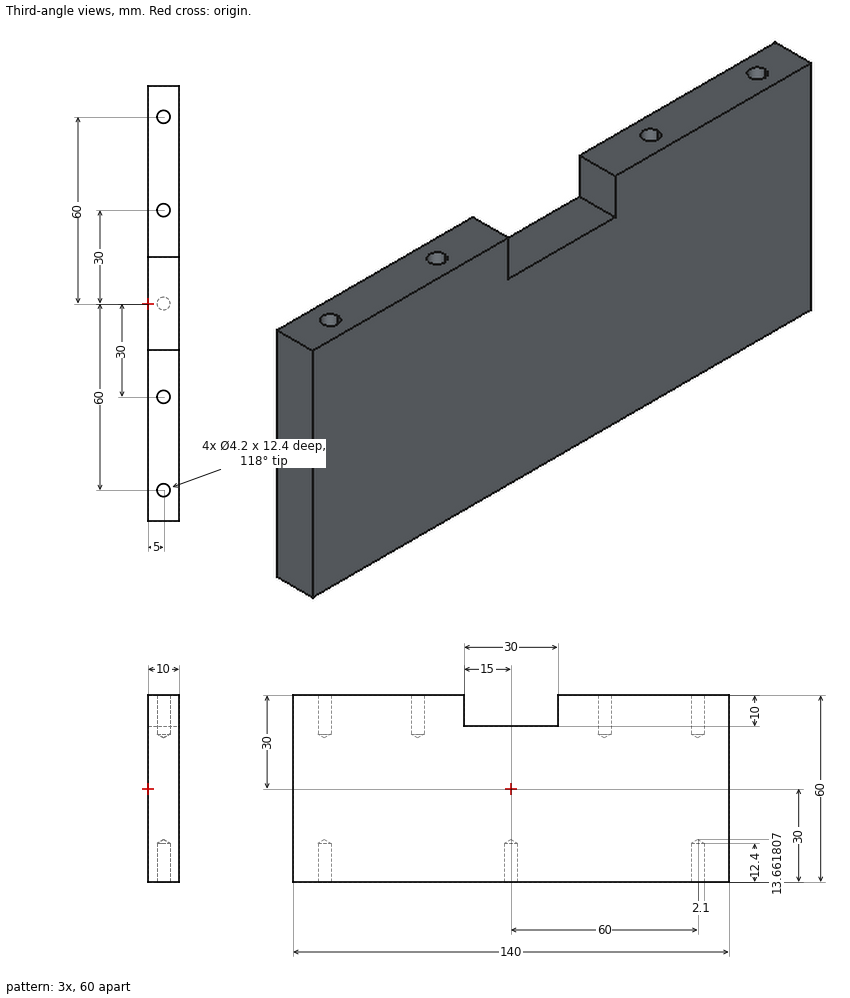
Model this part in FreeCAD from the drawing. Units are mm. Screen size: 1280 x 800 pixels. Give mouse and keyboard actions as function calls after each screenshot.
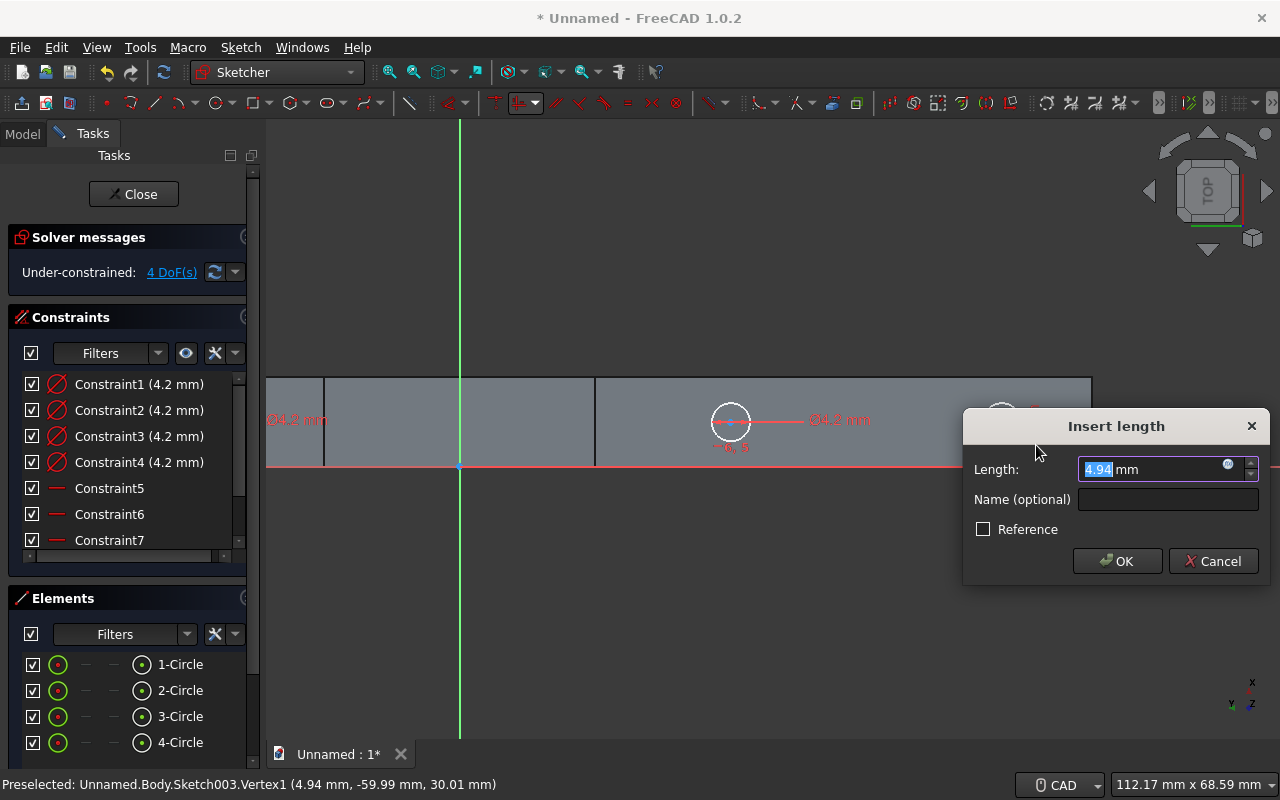
text(5)
key(Return)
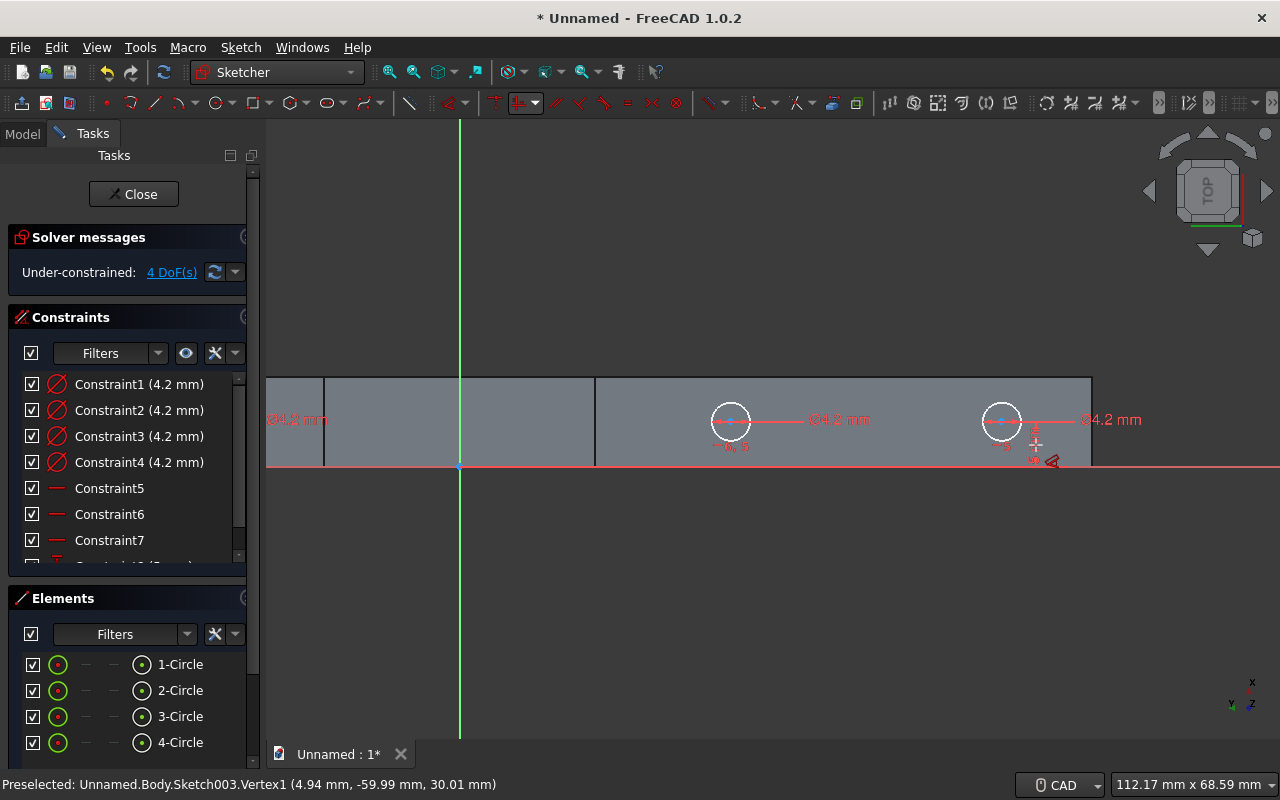
click(1002, 422)
click(731, 501)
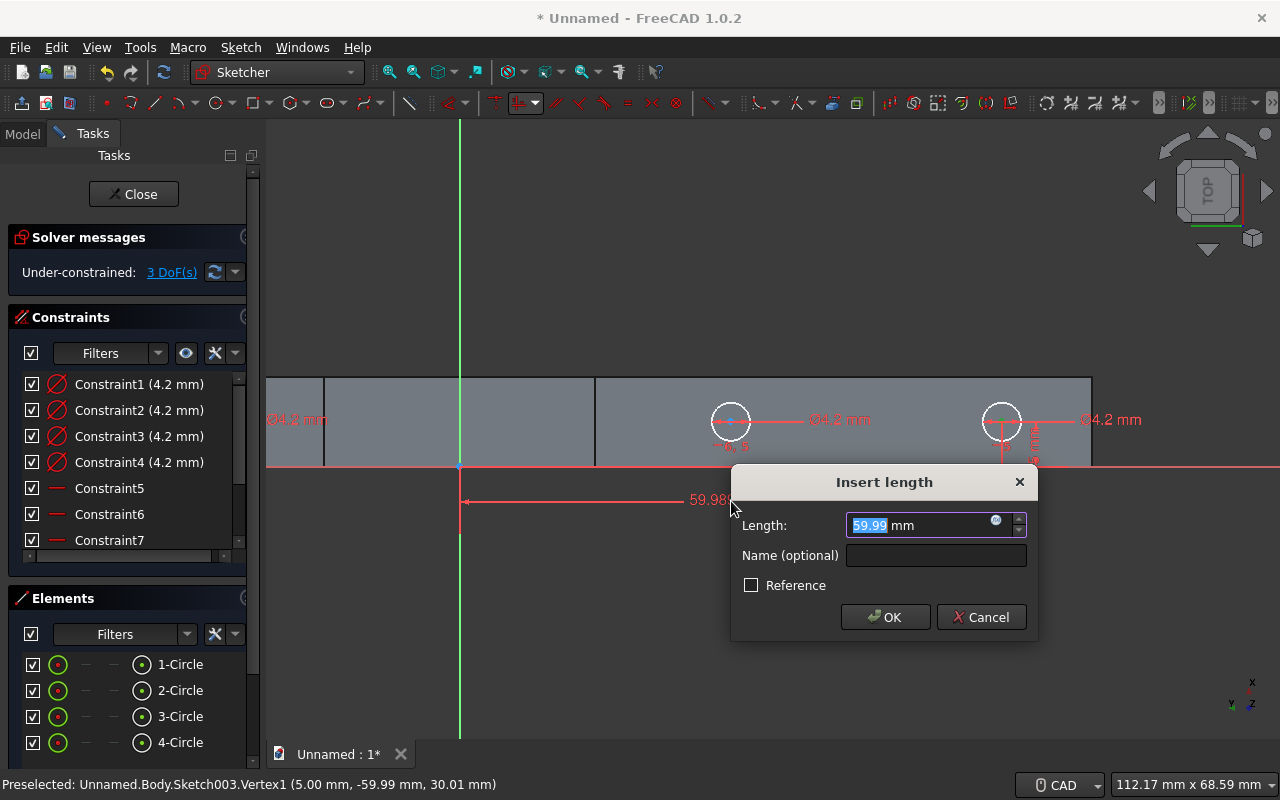
text(60)
key(Return)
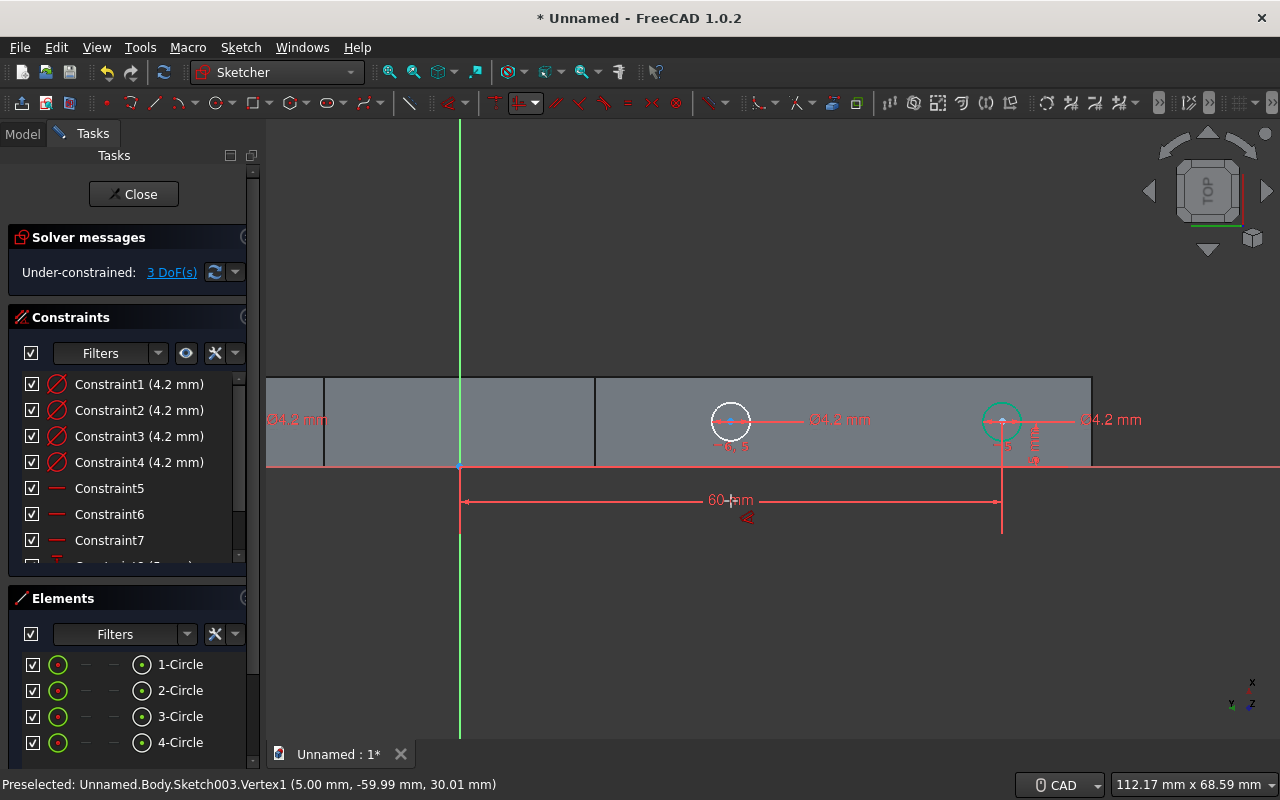
click(731, 422)
click(595, 501)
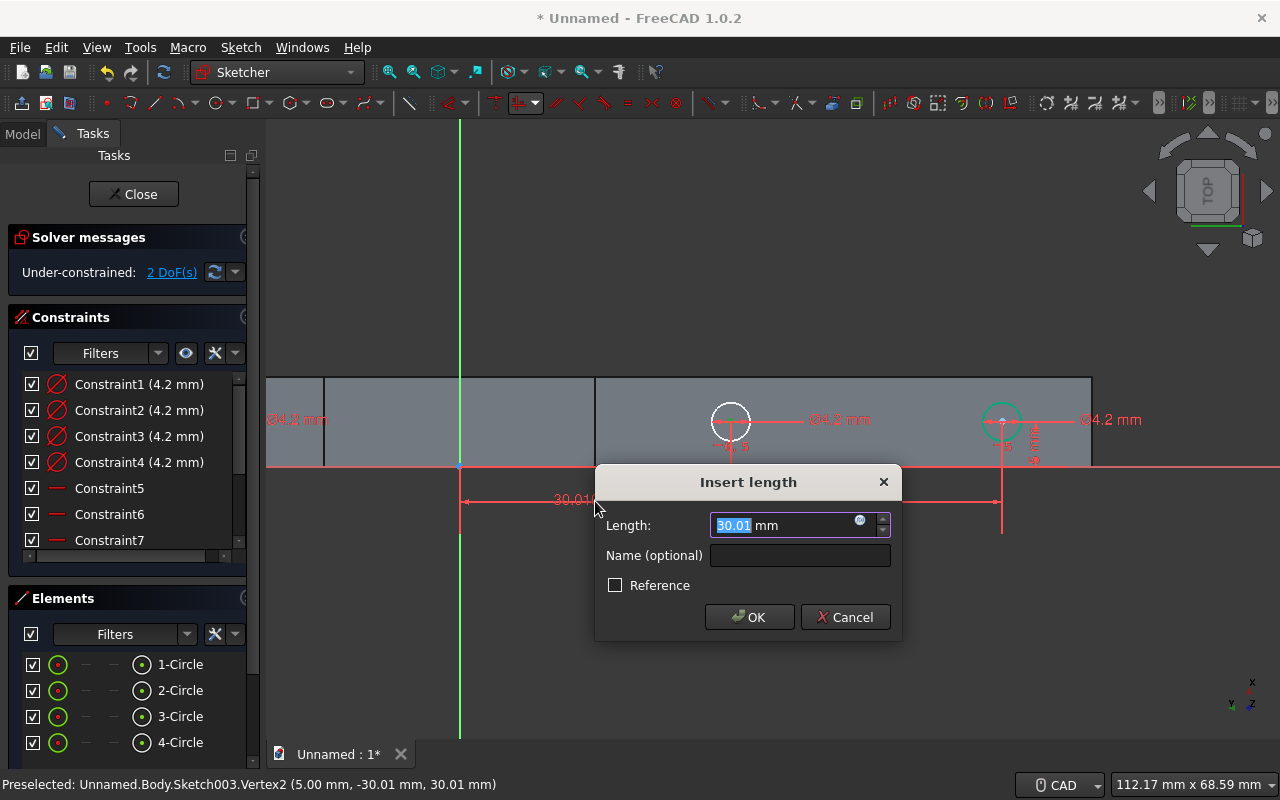
text(30)
key(Return)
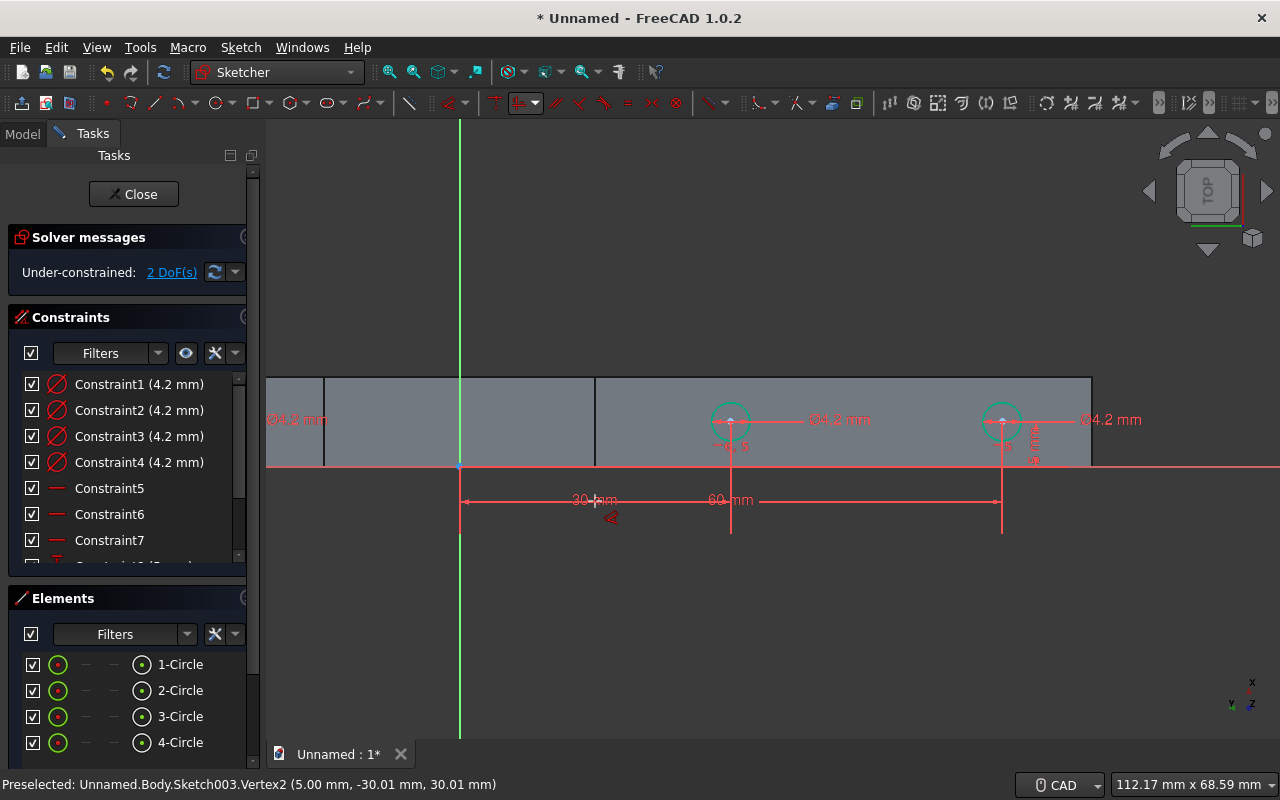
scroll(1002, 422, down, 3)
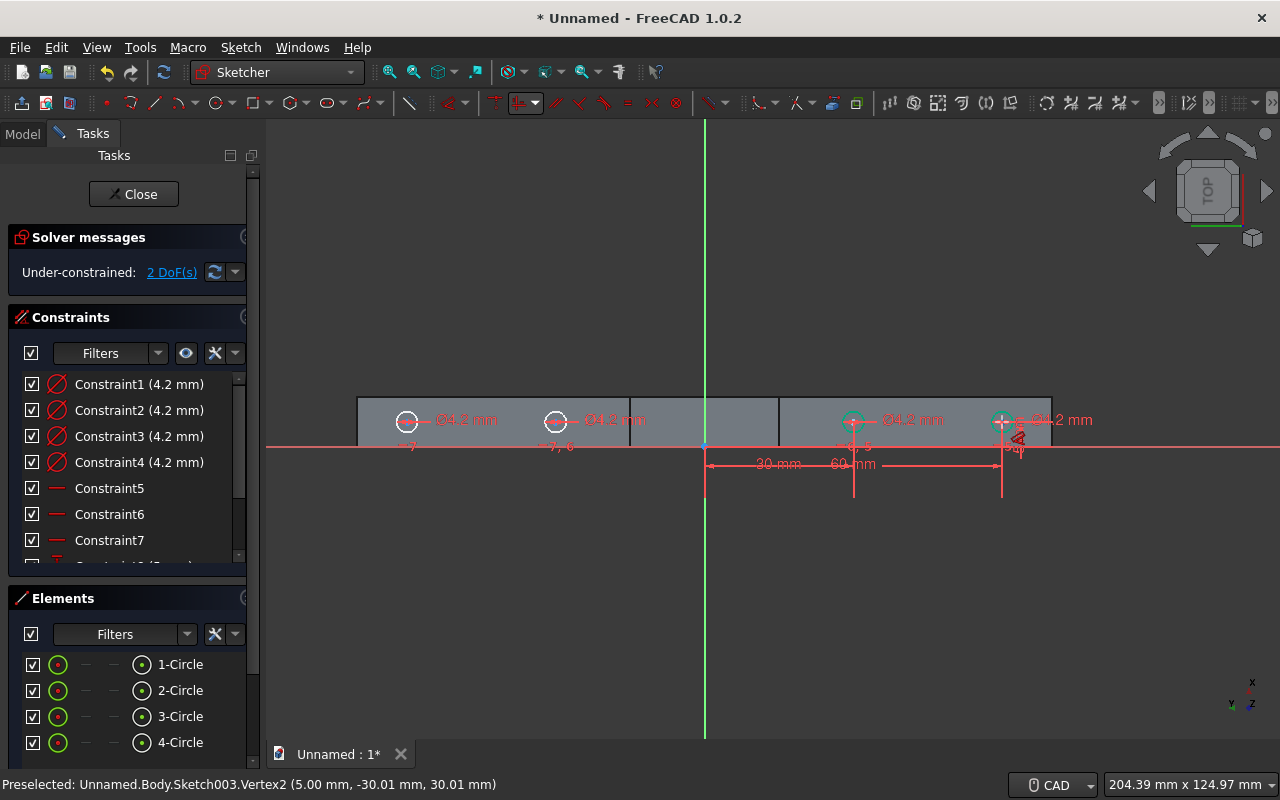
click(556, 422)
click(630, 481)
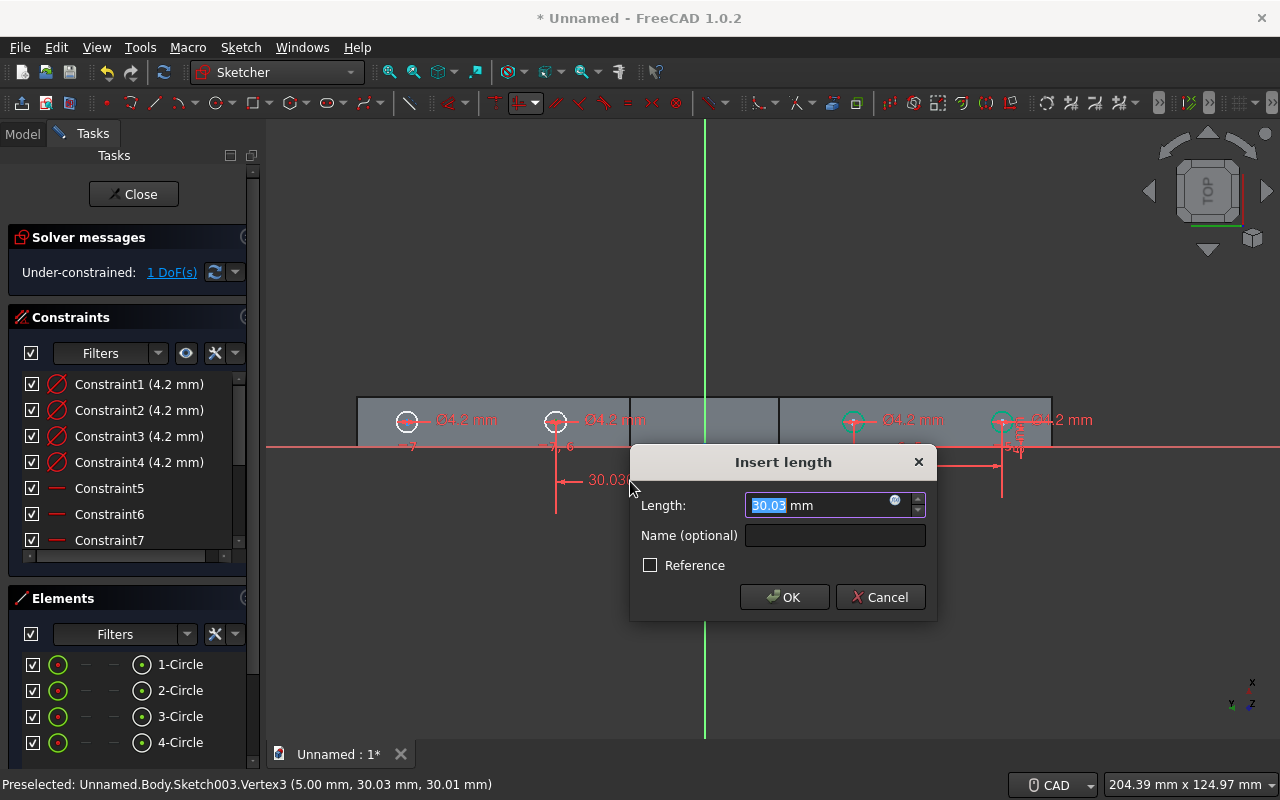
text(30)
key(Return)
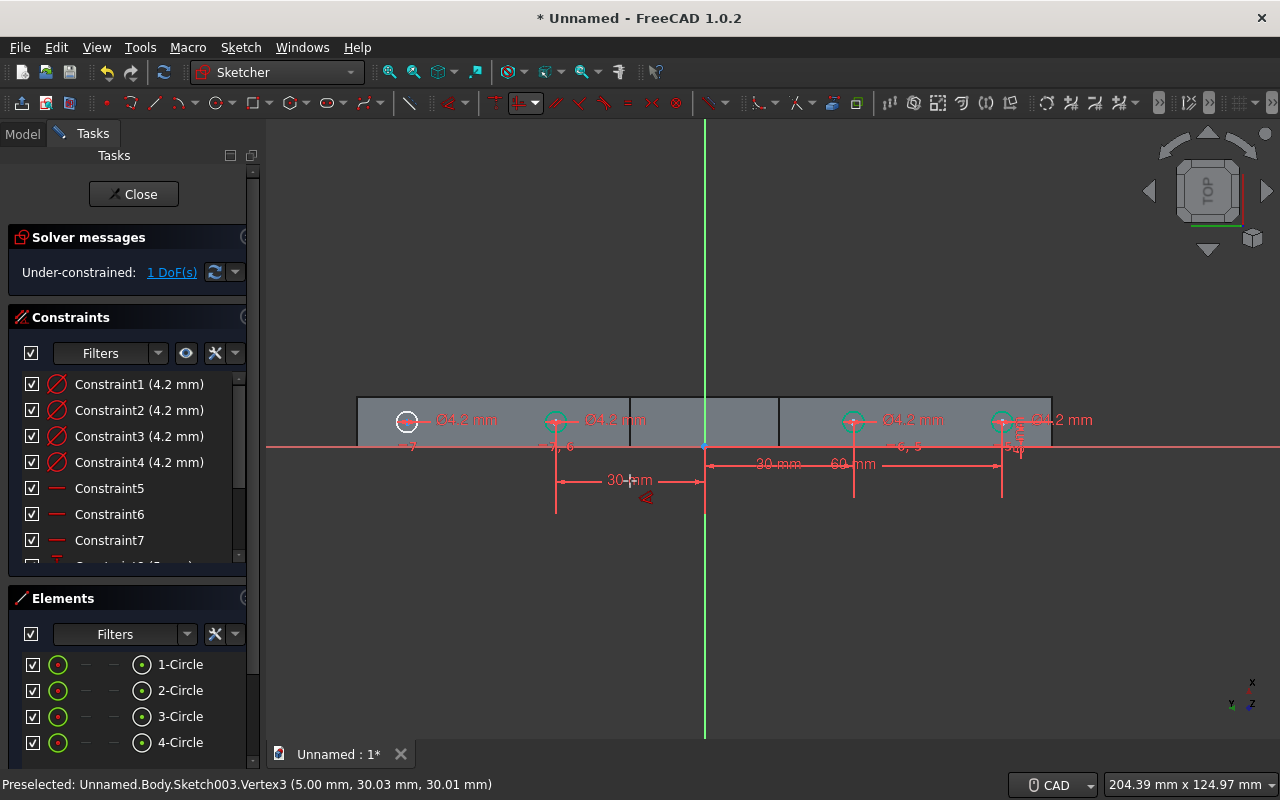
click(407, 422)
click(556, 481)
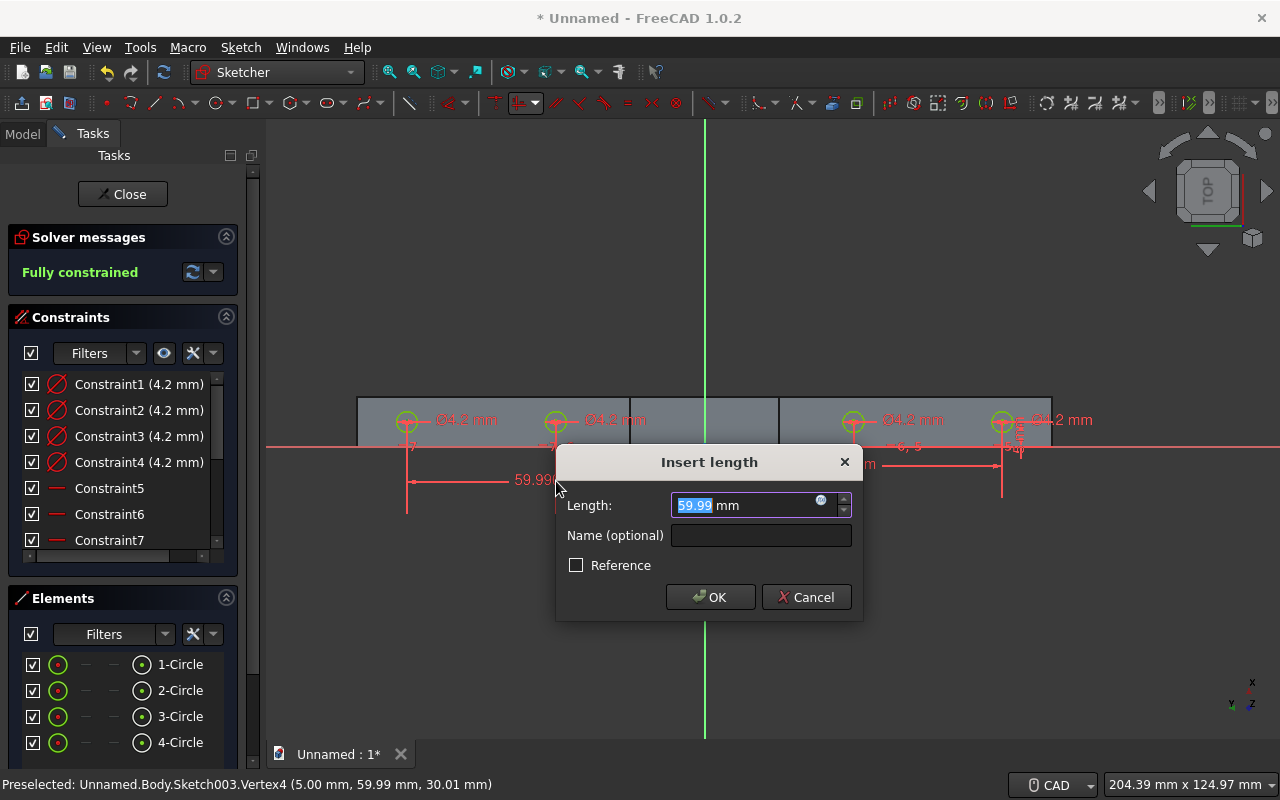
text(60)
key(Return)
key(Escape)